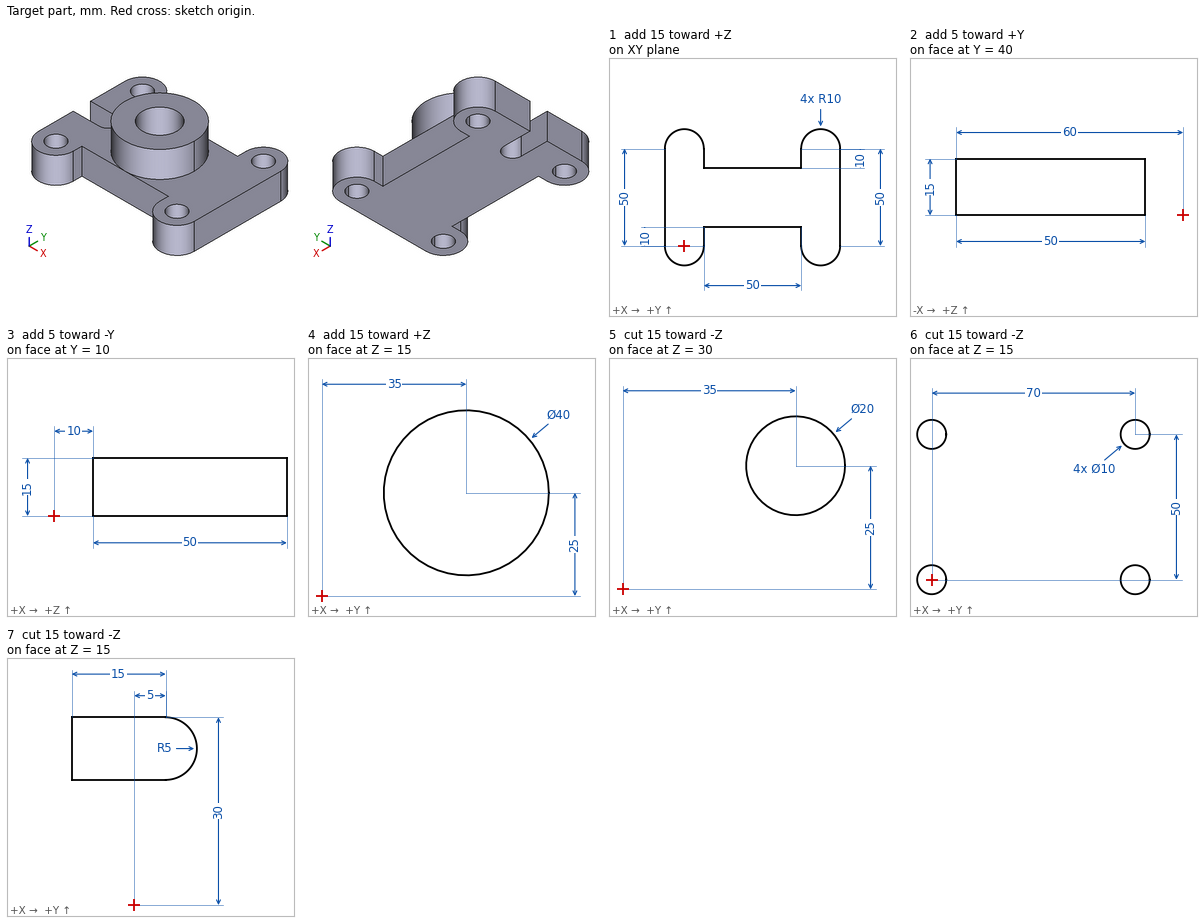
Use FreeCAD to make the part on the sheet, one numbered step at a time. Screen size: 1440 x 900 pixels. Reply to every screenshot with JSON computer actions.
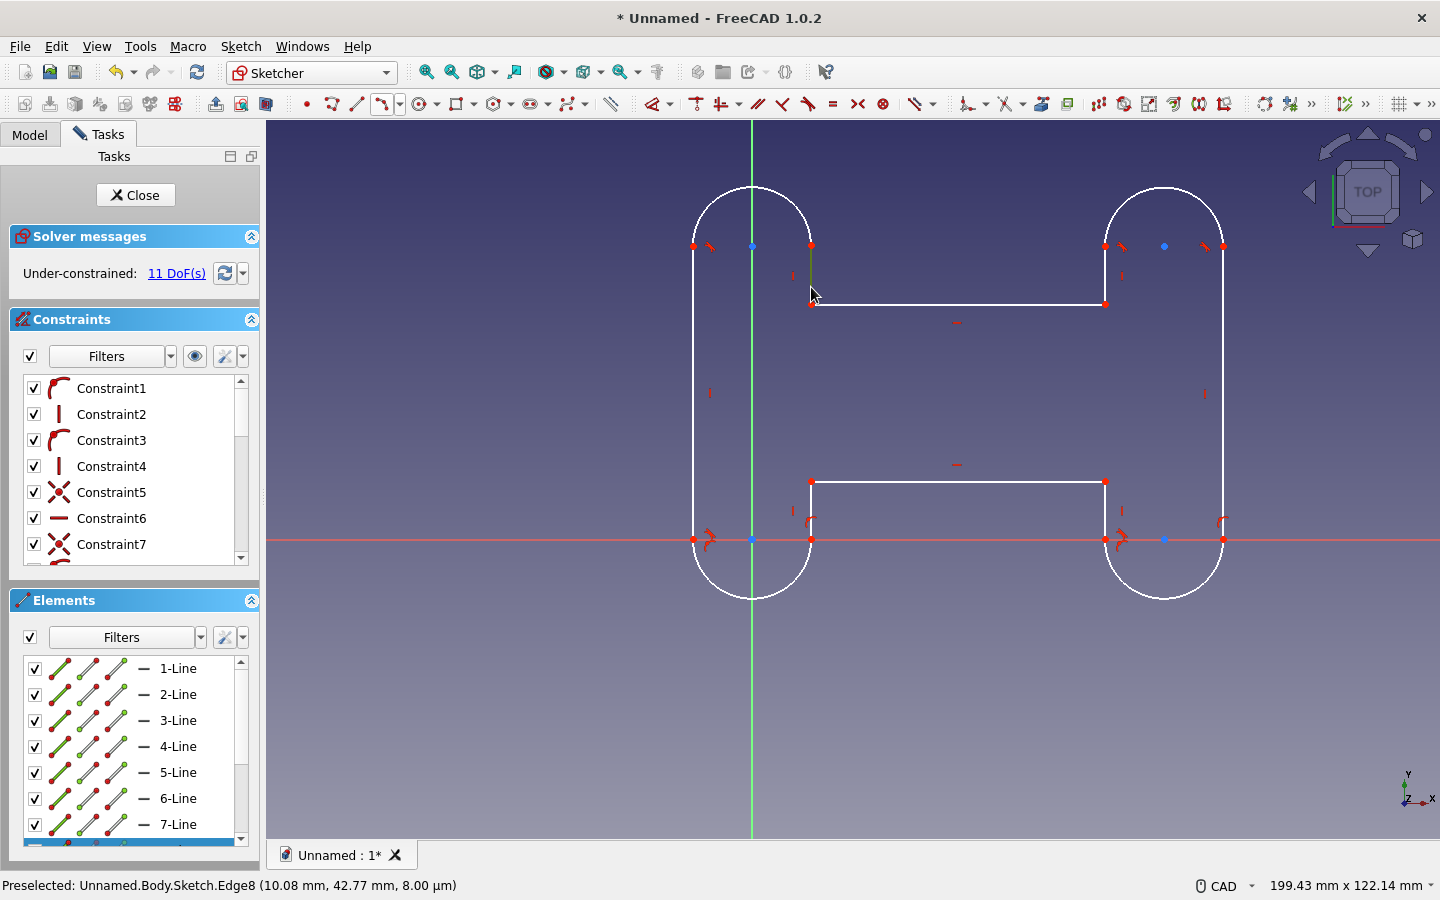
{"action": "left_click", "coordinate": [787, 198]}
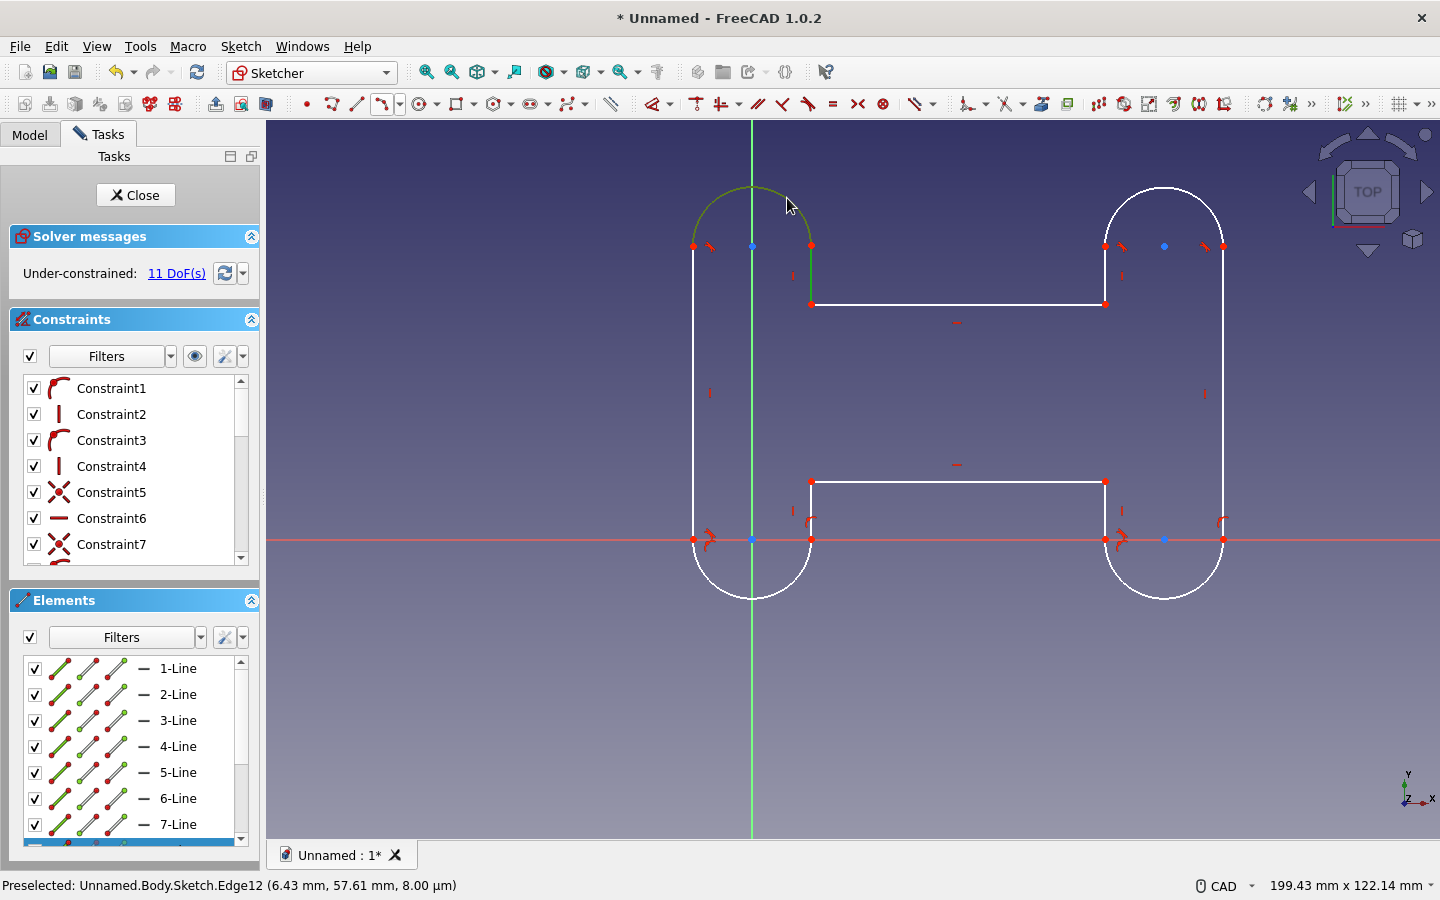
{"action": "left_click", "coordinate": [808, 104]}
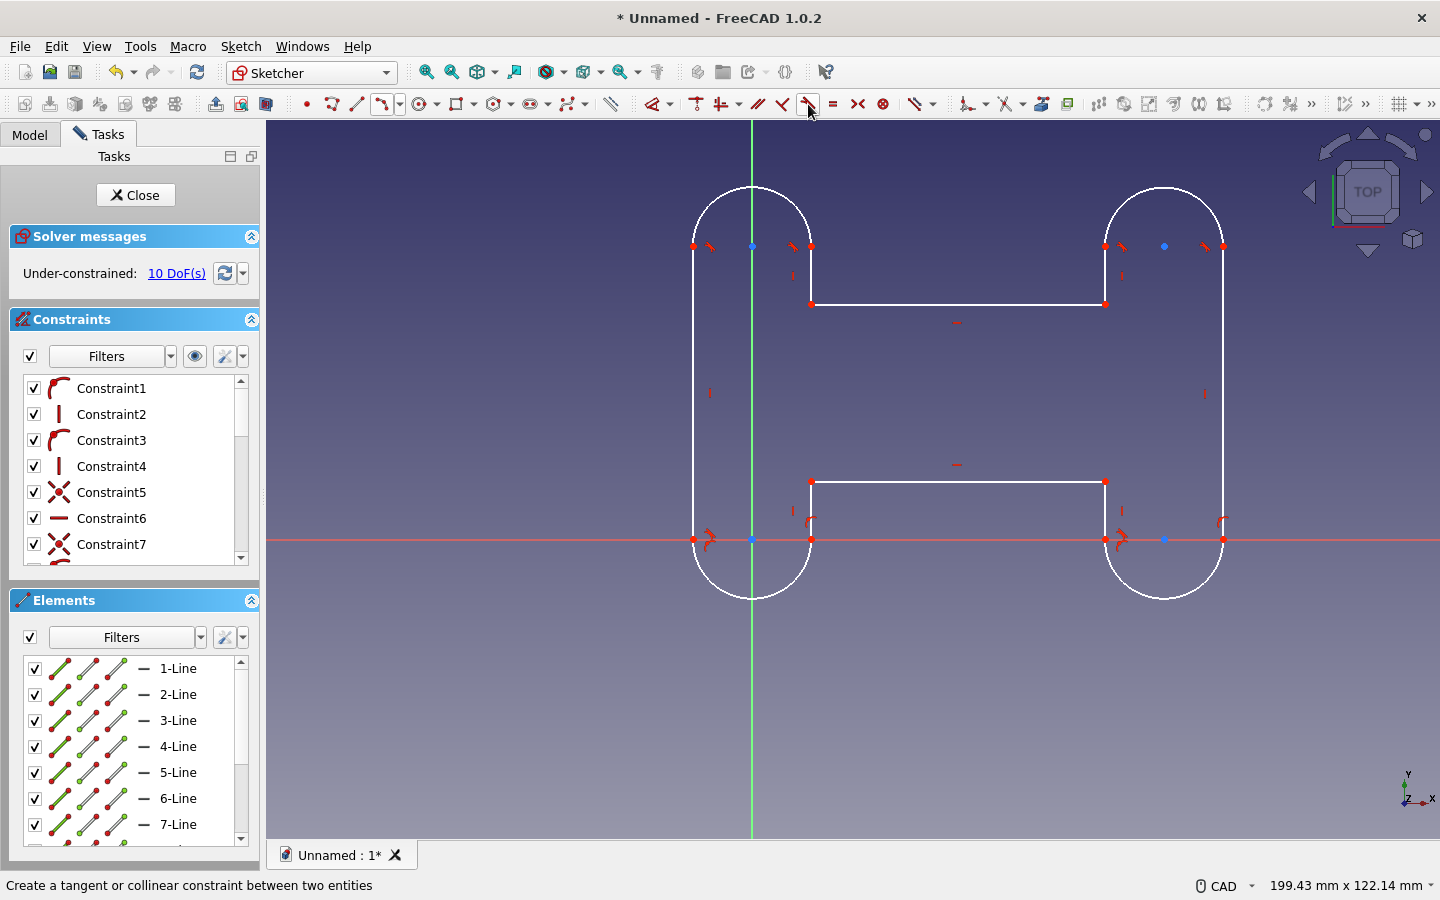
{"action": "left_click", "coordinate": [717, 587]}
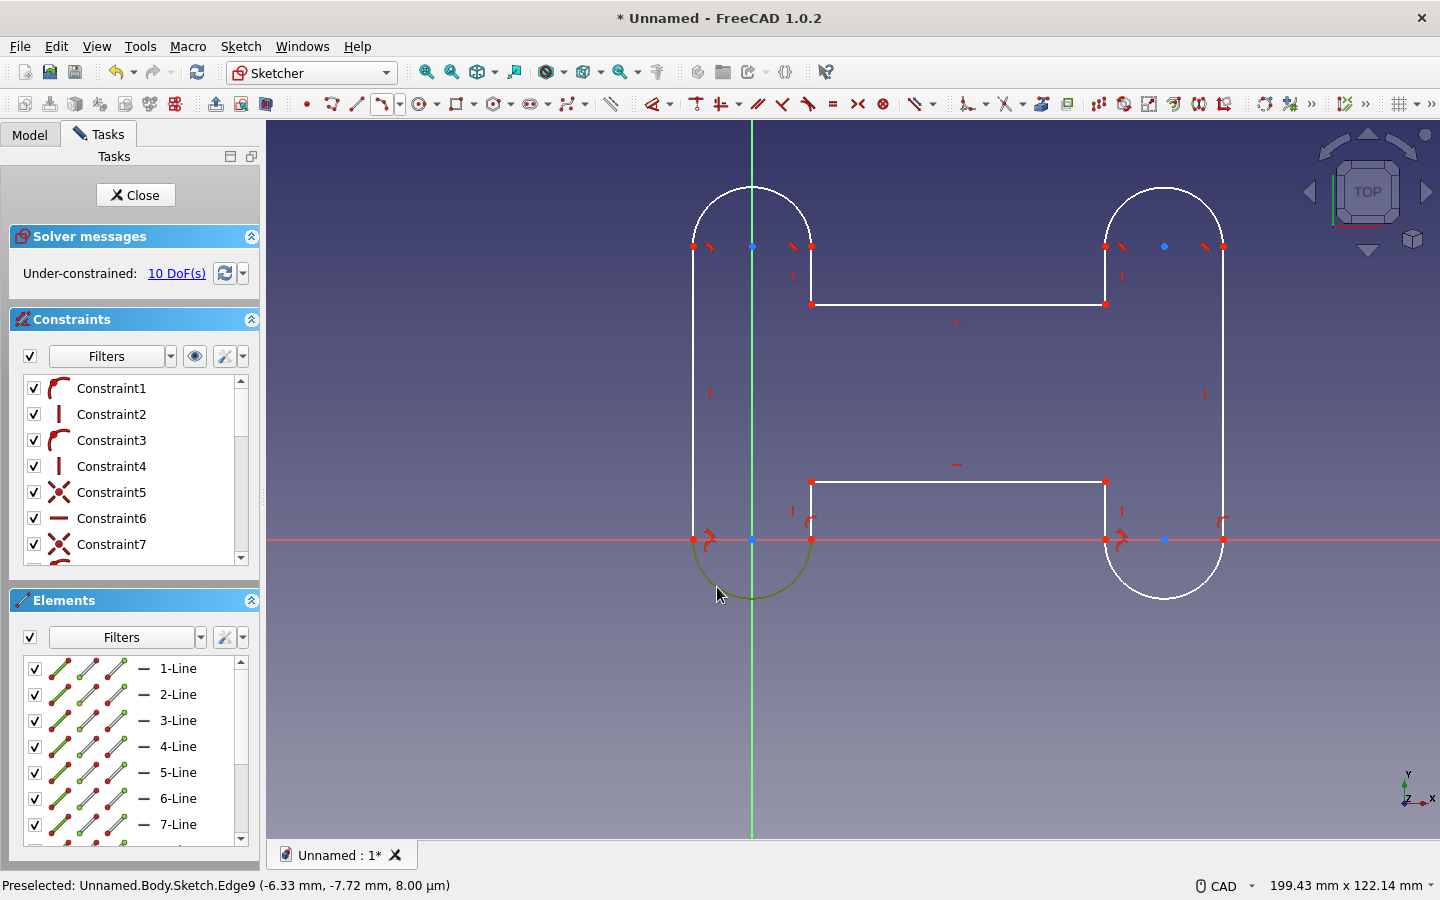
{"action": "left_click", "coordinate": [1129, 587]}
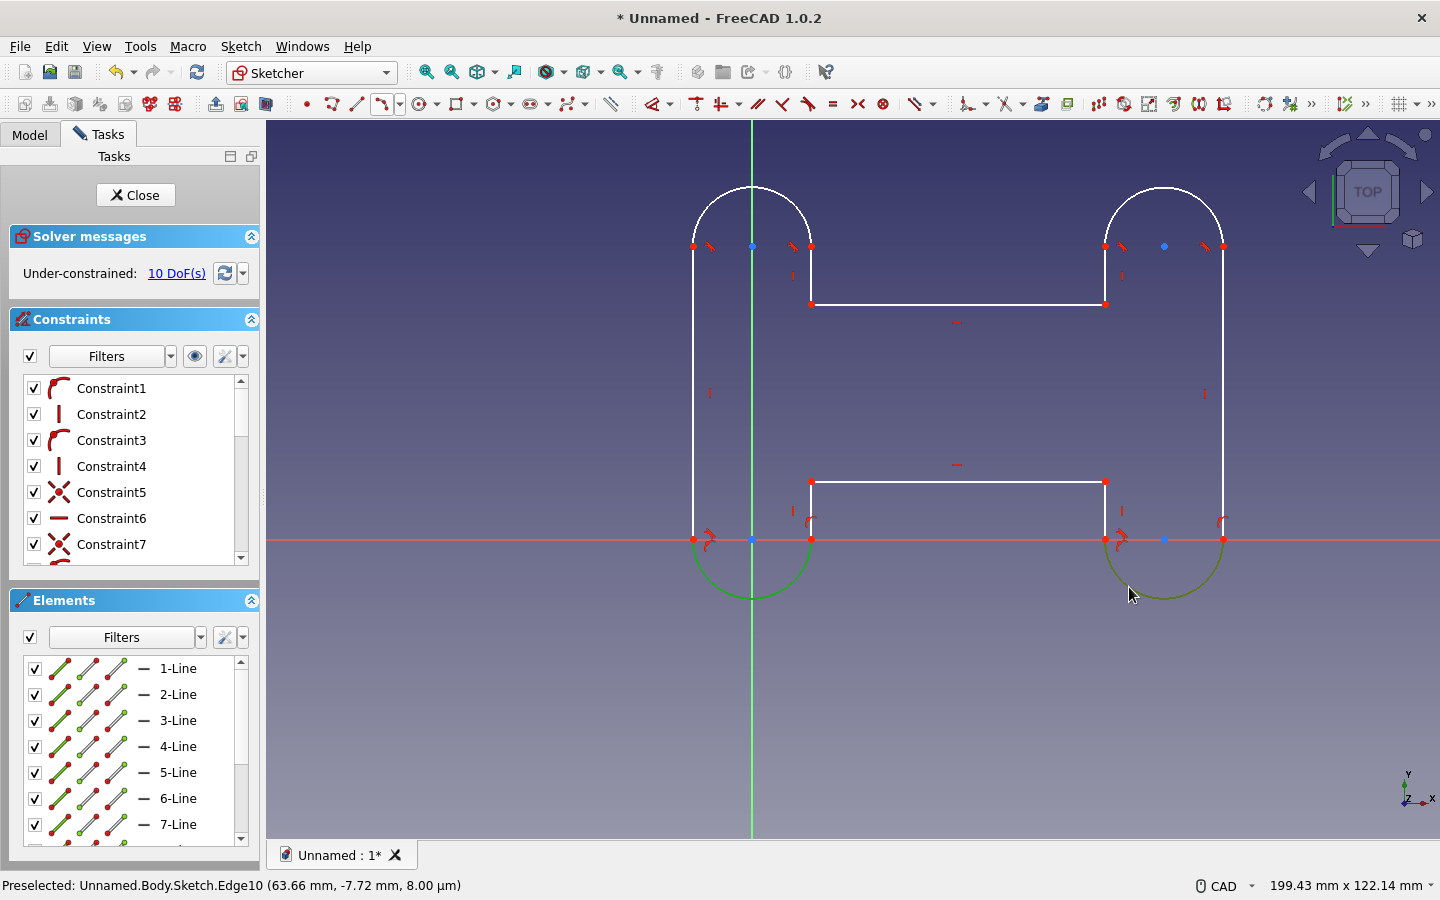
{"action": "left_click", "coordinate": [1199, 199]}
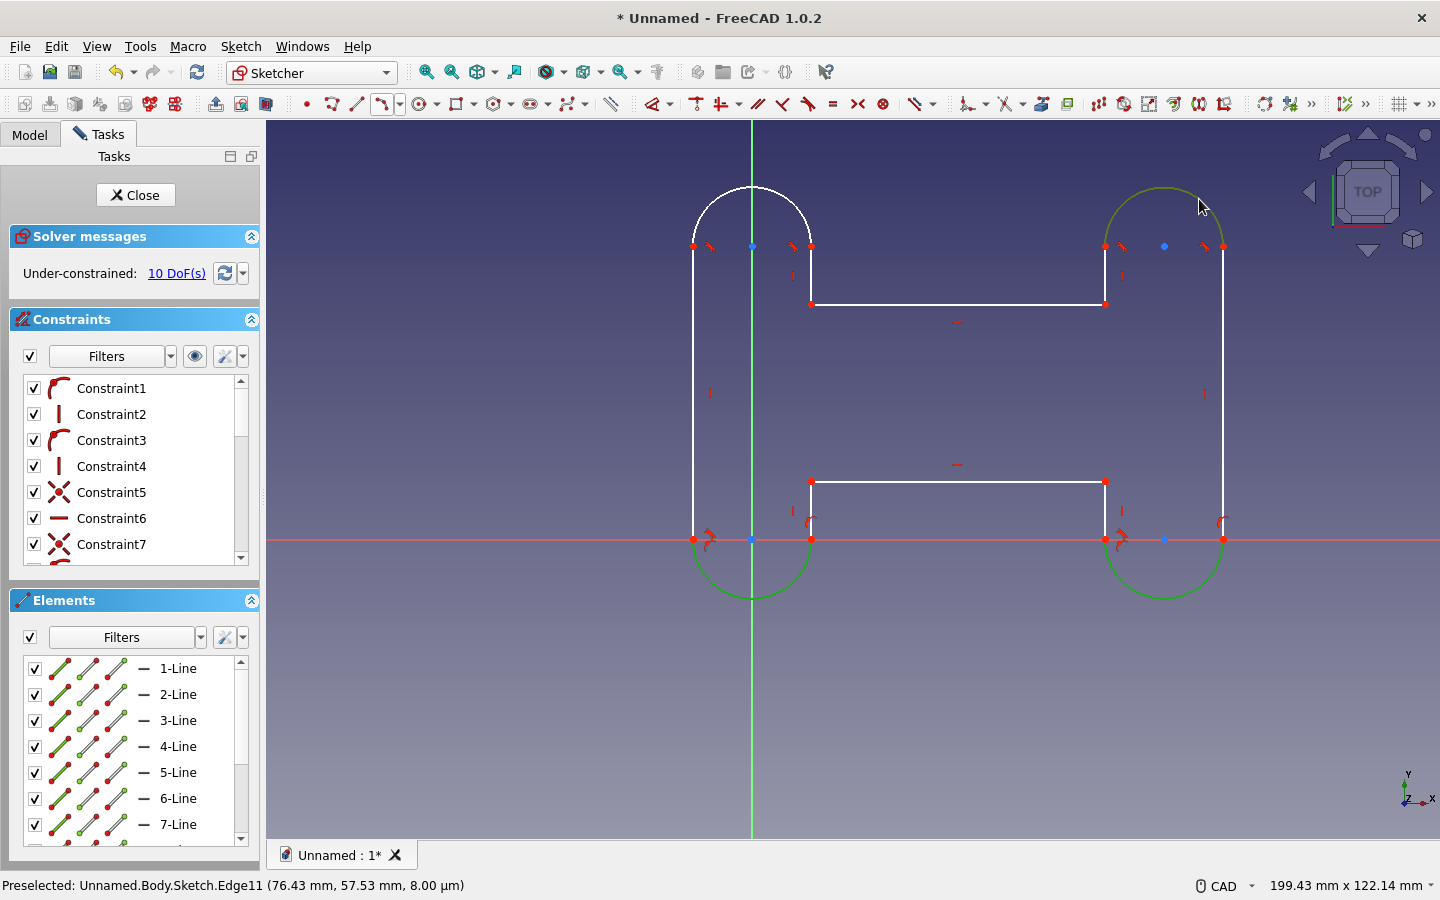
{"action": "left_click", "coordinate": [787, 198]}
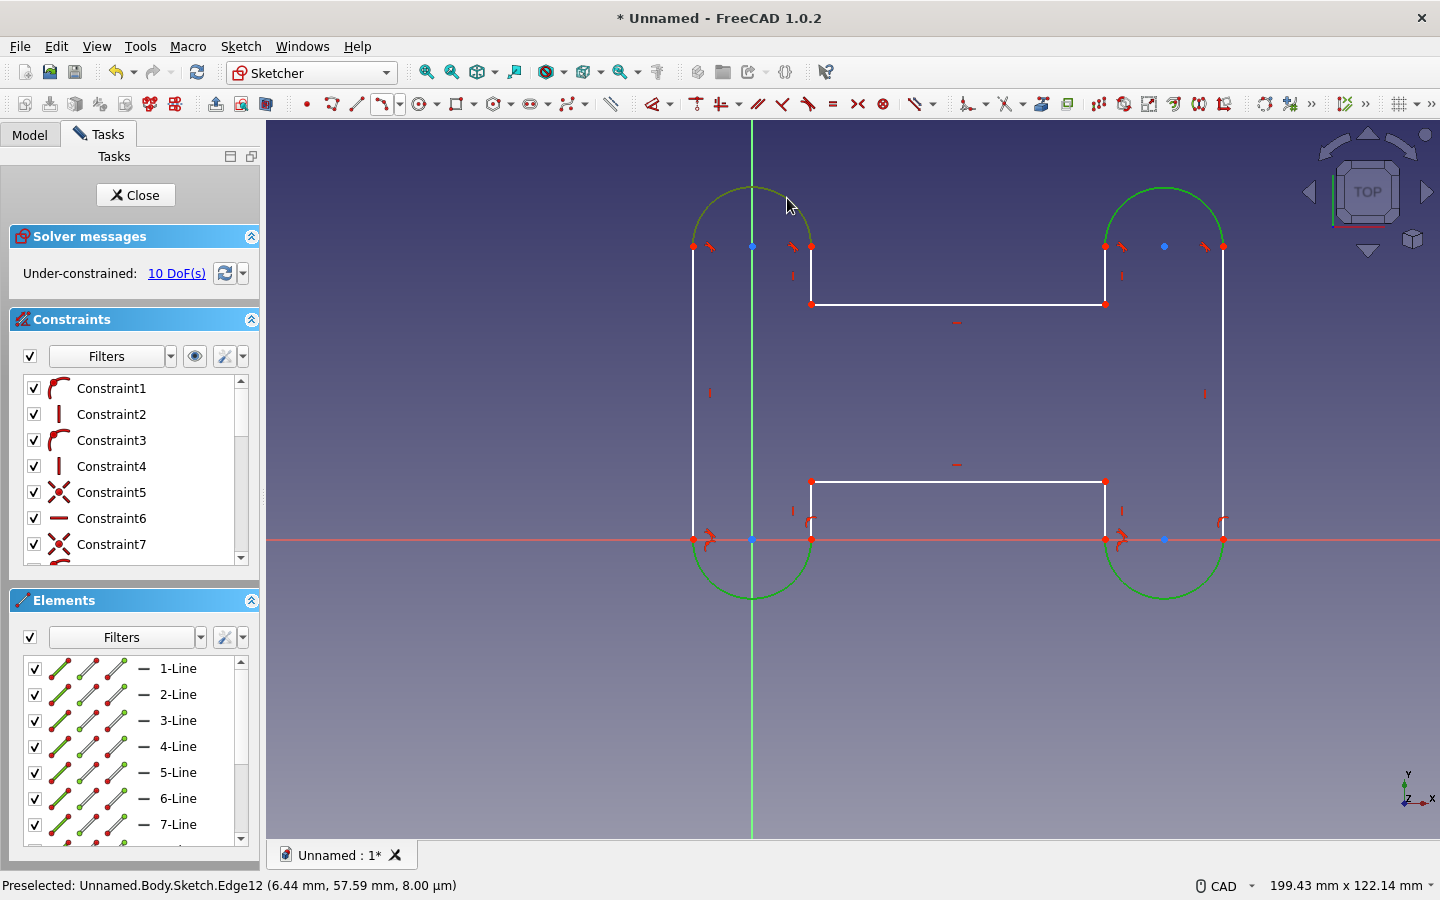
{"action": "left_click", "coordinate": [833, 104]}